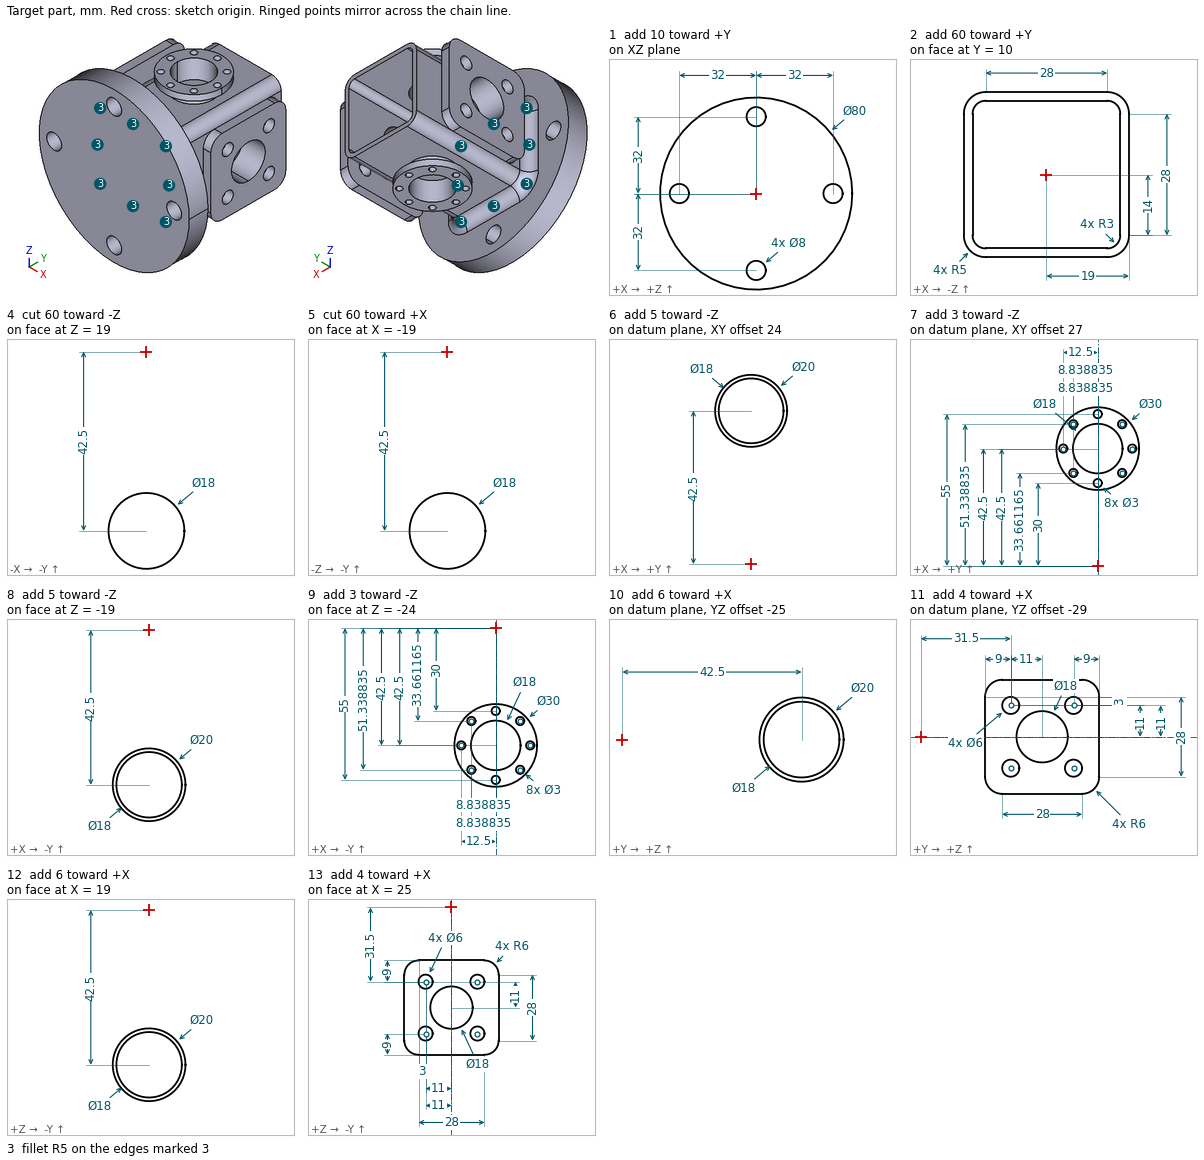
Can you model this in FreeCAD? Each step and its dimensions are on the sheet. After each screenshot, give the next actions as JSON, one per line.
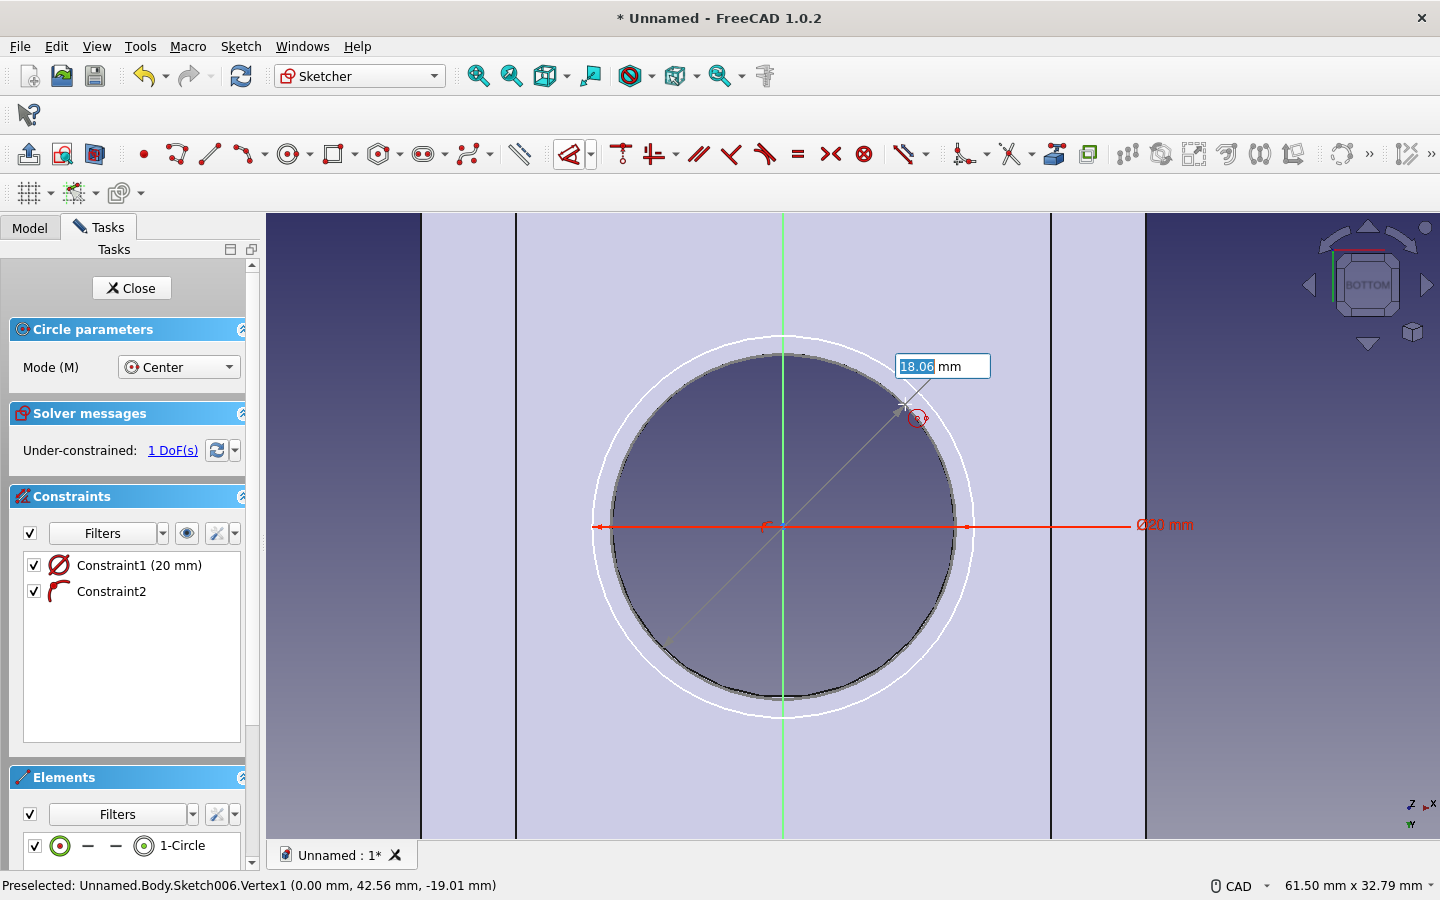
{"action": "type", "text": "18"}
{"action": "key", "text": "Return"}
{"action": "key", "text": "Escape"}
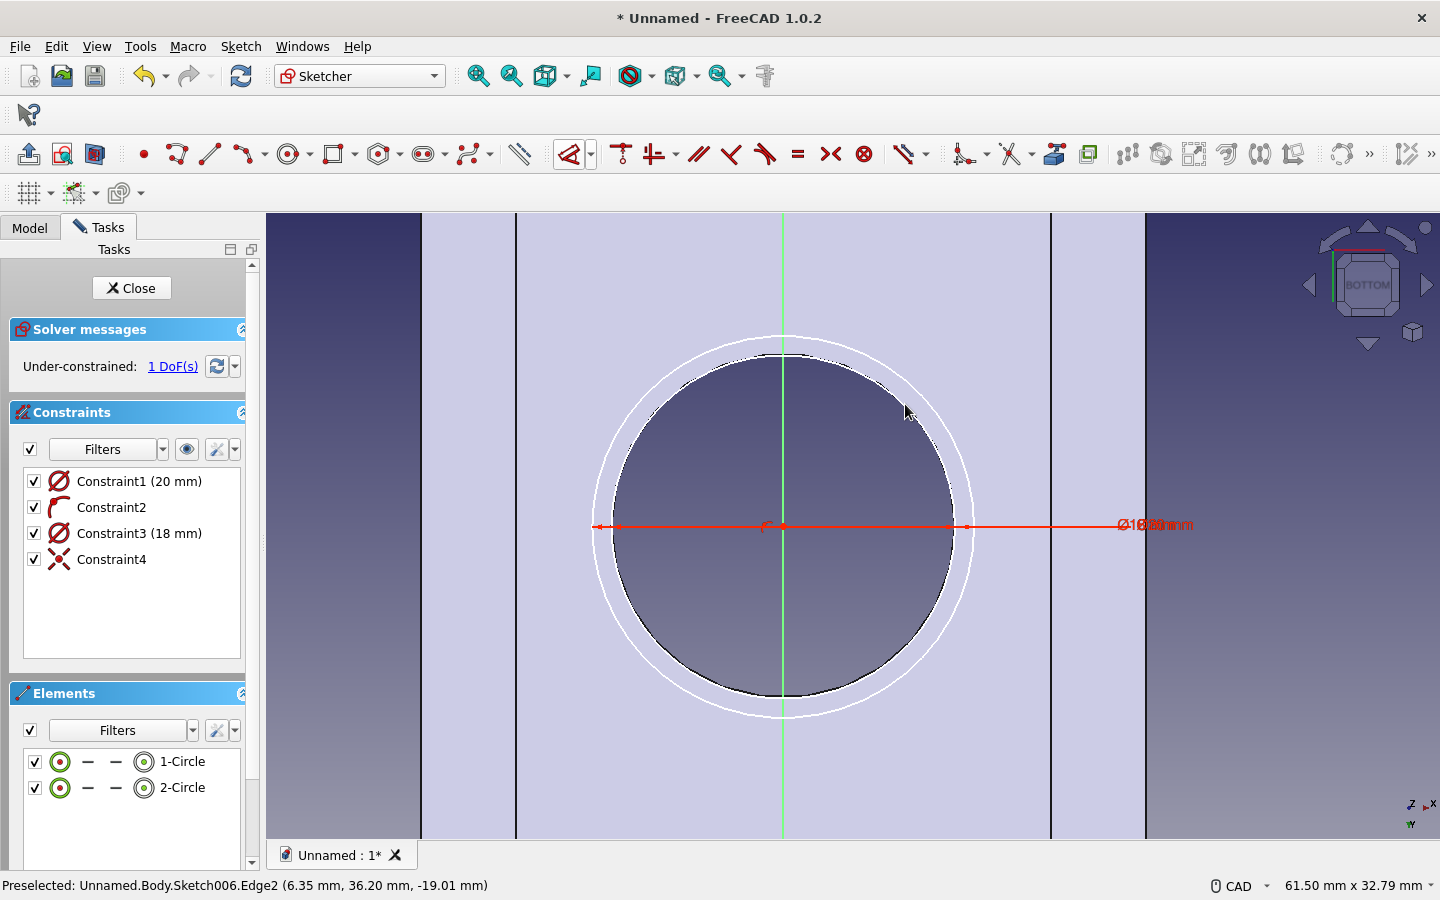
{"action": "left_click", "coordinate": [783, 527]}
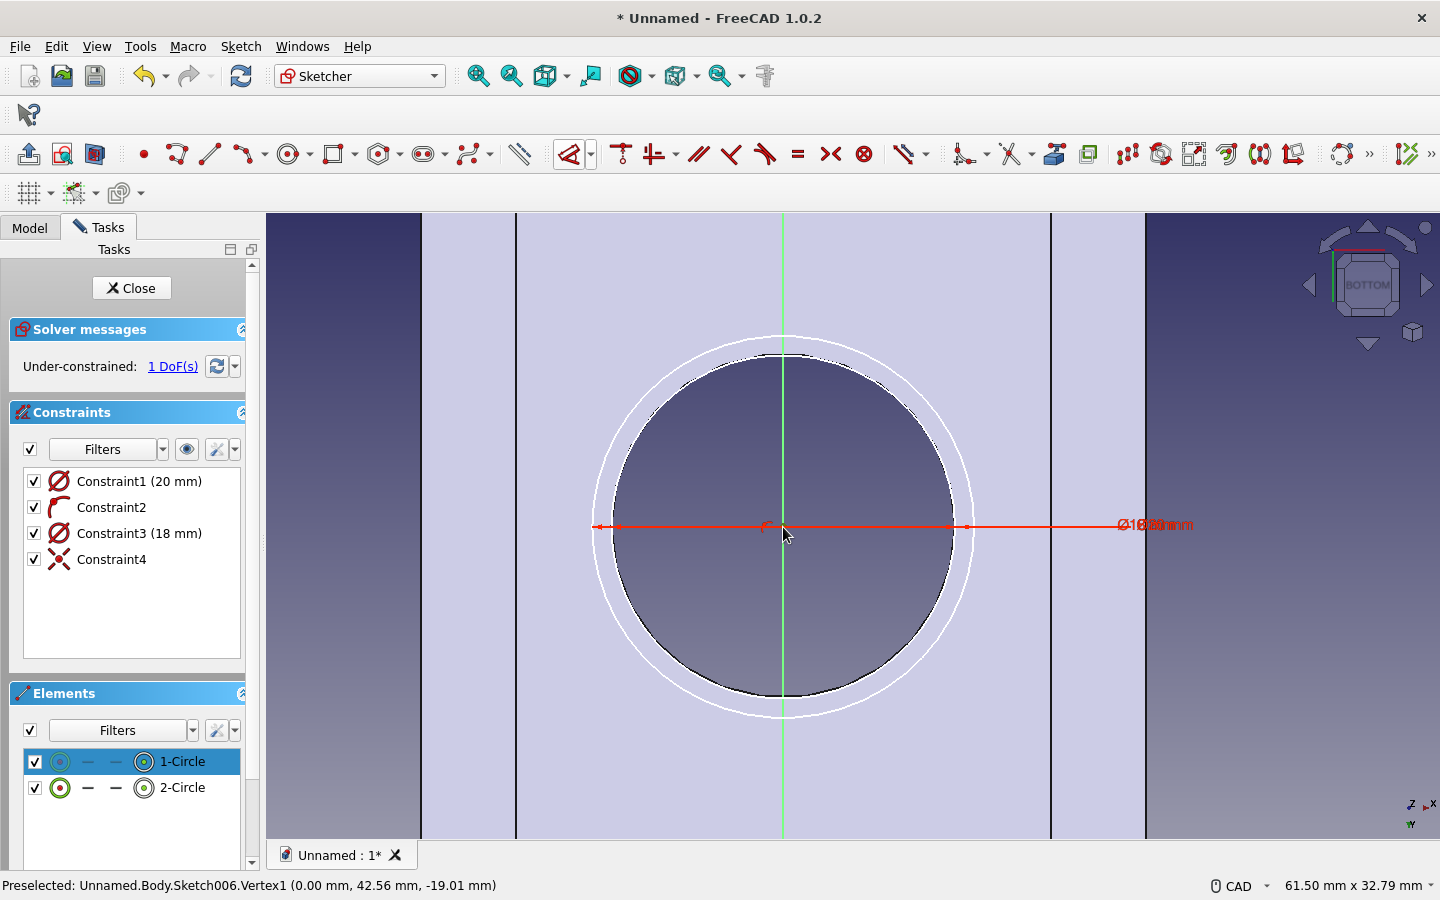
{"action": "key", "text": "i"}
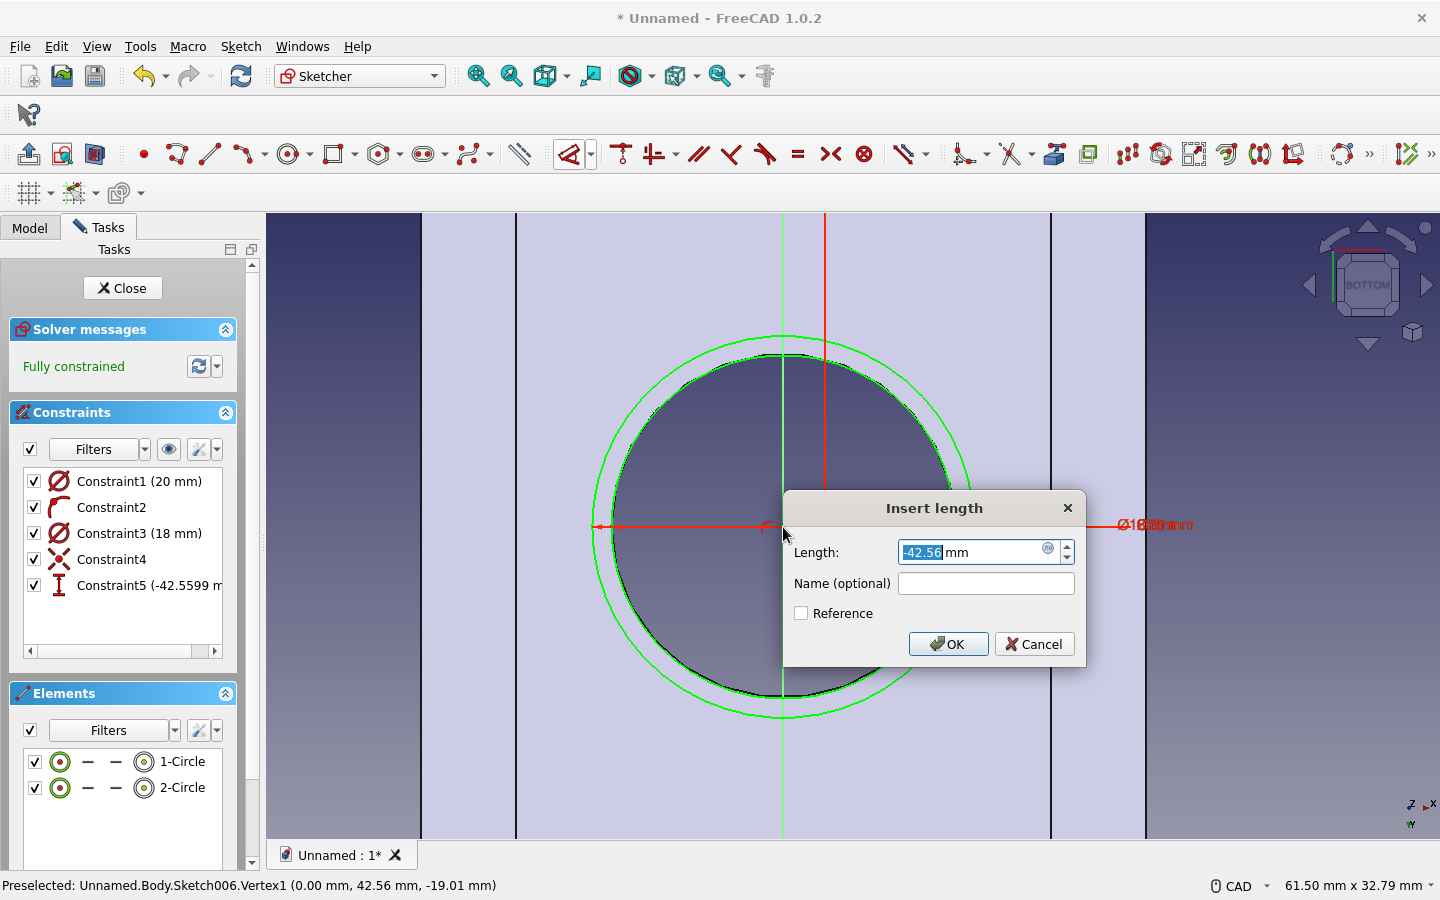
{"action": "type", "text": "-42.5"}
{"action": "key", "text": "Return"}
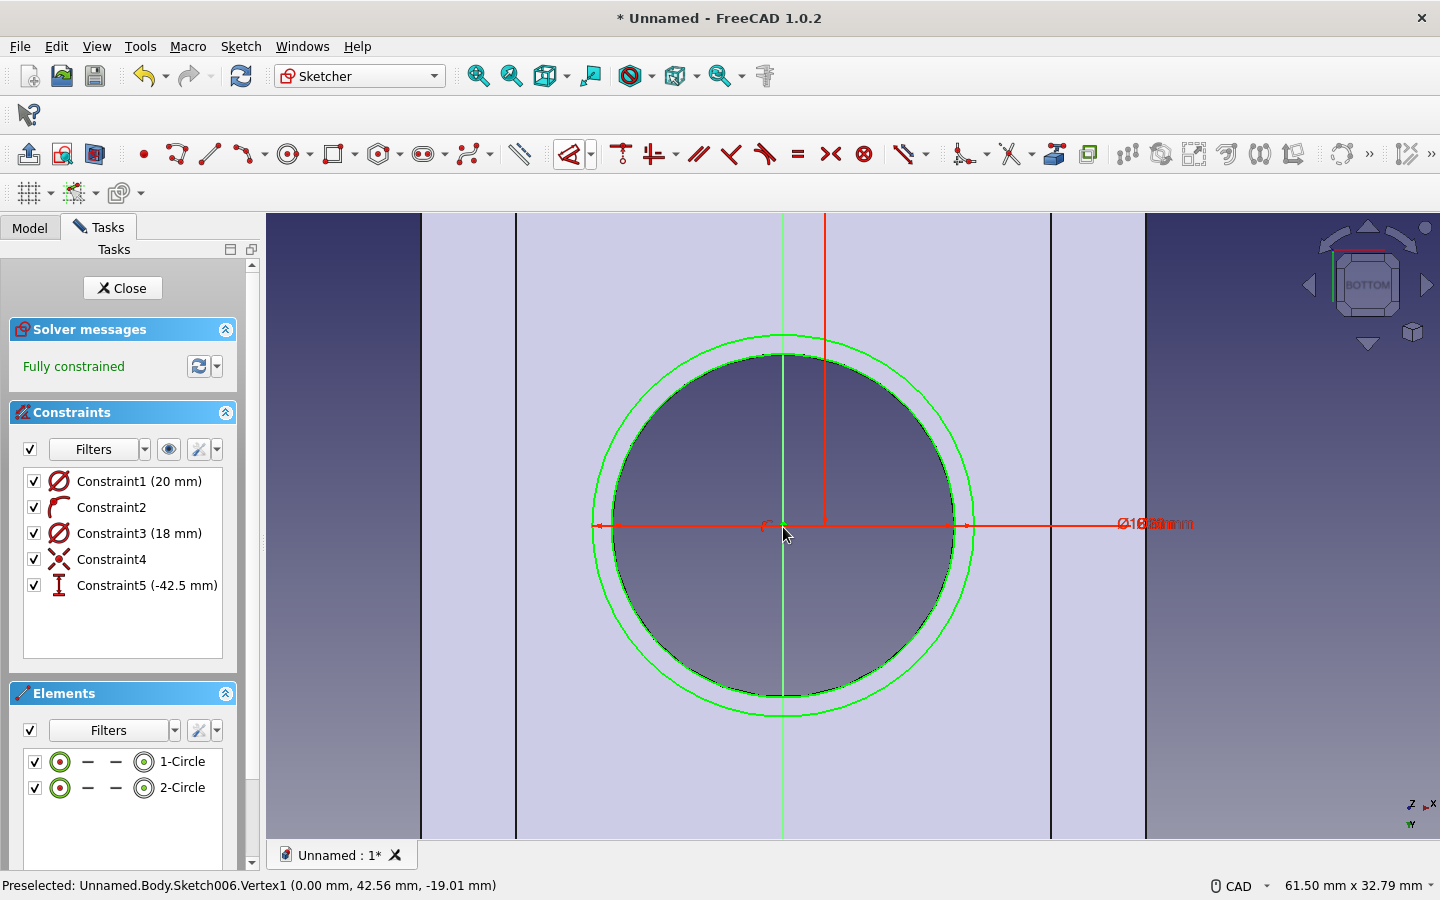
{"action": "left_click", "coordinate": [123, 288]}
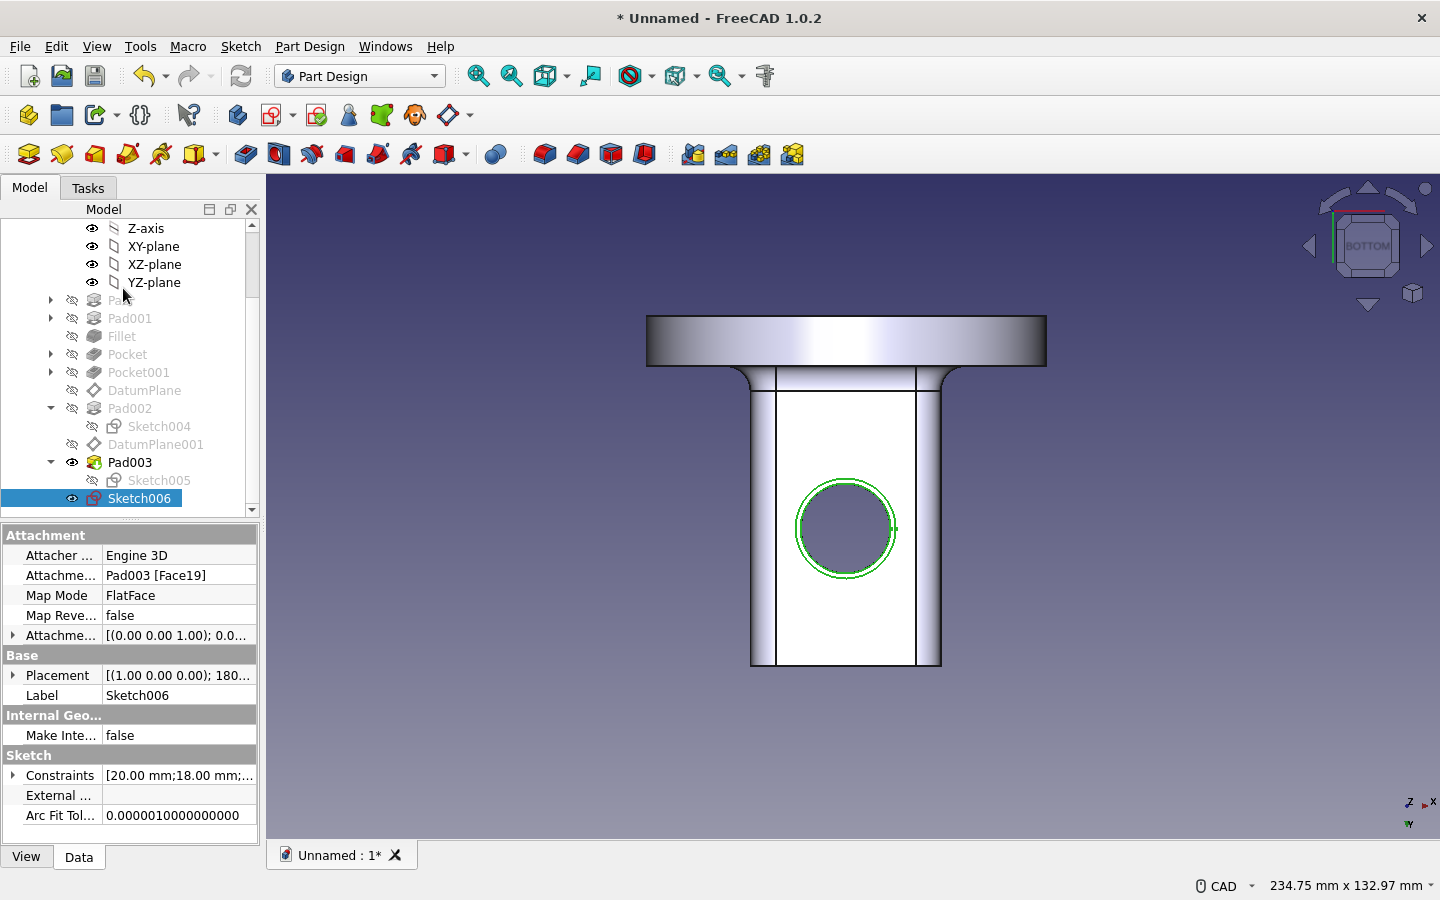
{"action": "left_click", "coordinate": [29, 154]}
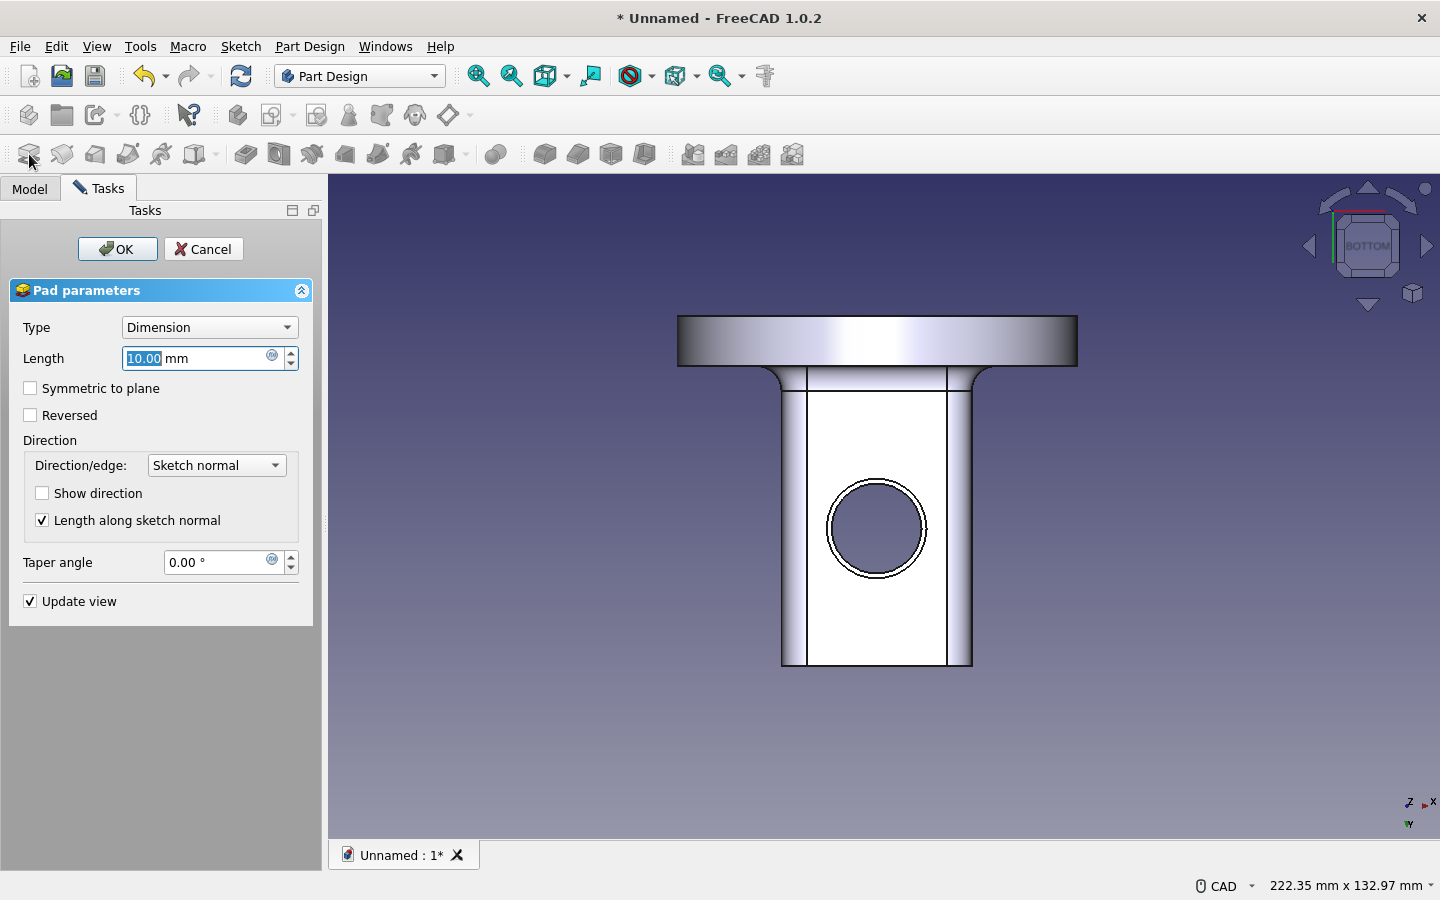
{"action": "type", "text": "5"}
{"action": "key", "text": "Tab"}